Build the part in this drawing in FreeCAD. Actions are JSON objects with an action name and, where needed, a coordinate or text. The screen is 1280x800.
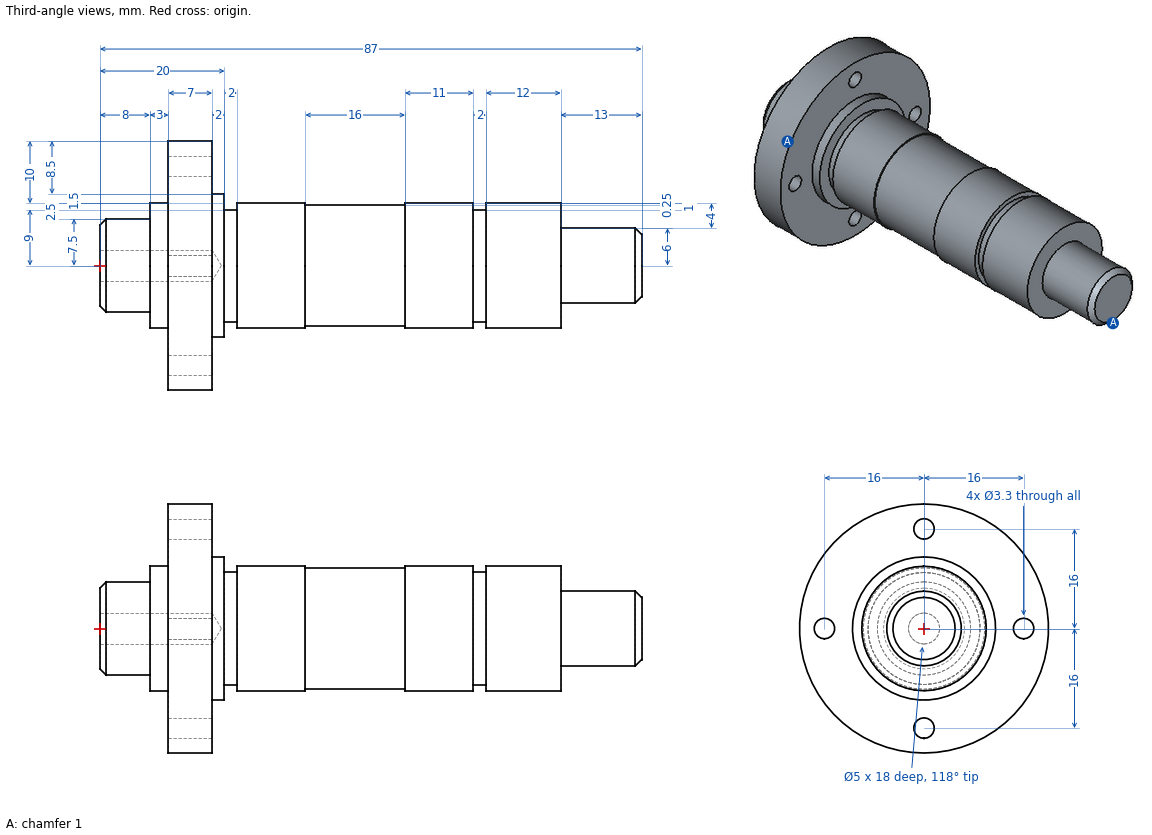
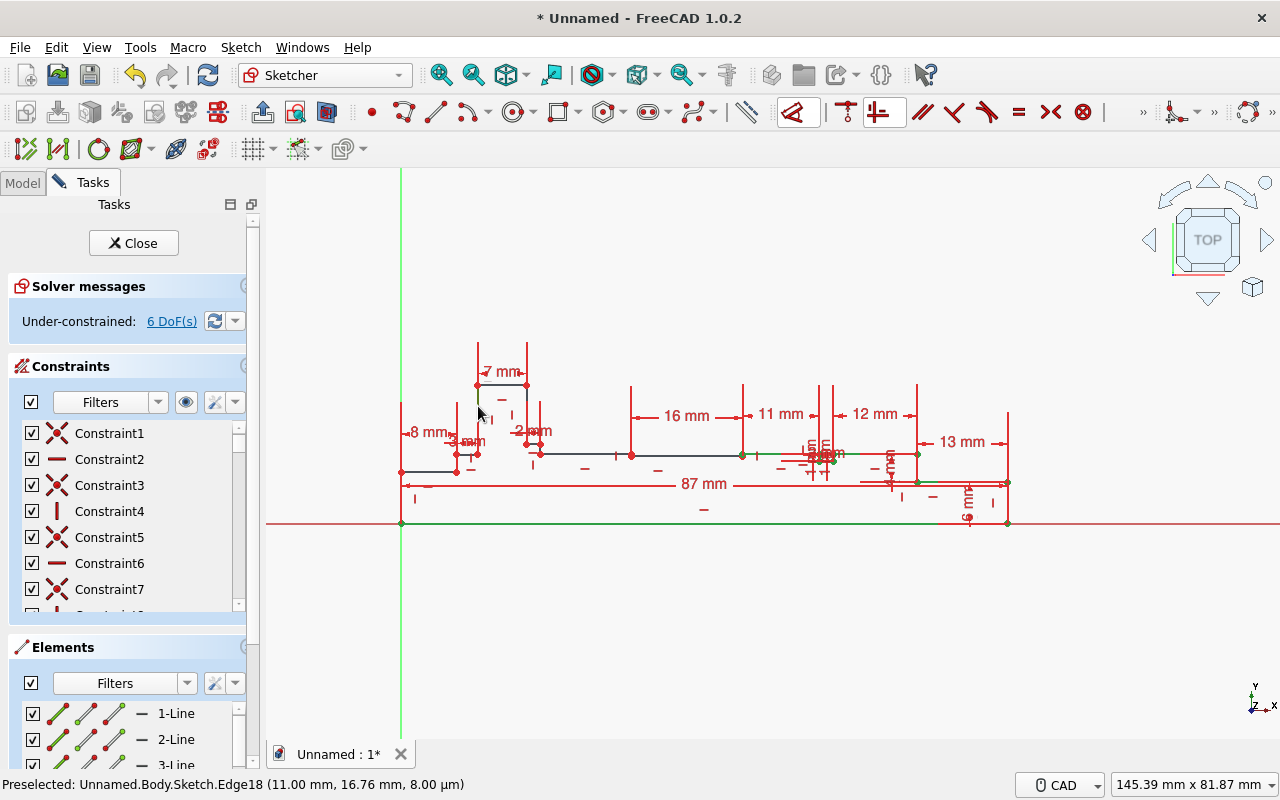
{"action": "key", "text": "i"}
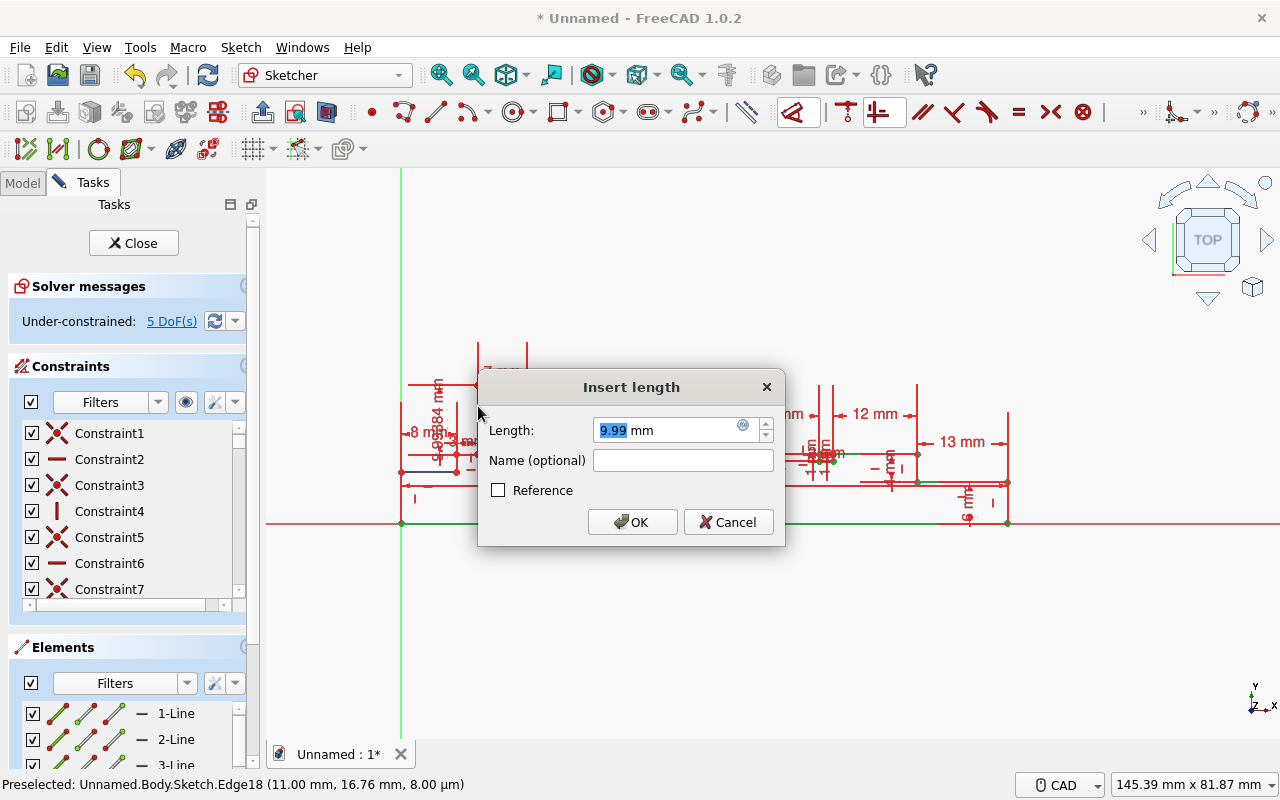
{"action": "type", "text": "10"}
{"action": "key", "text": "Return"}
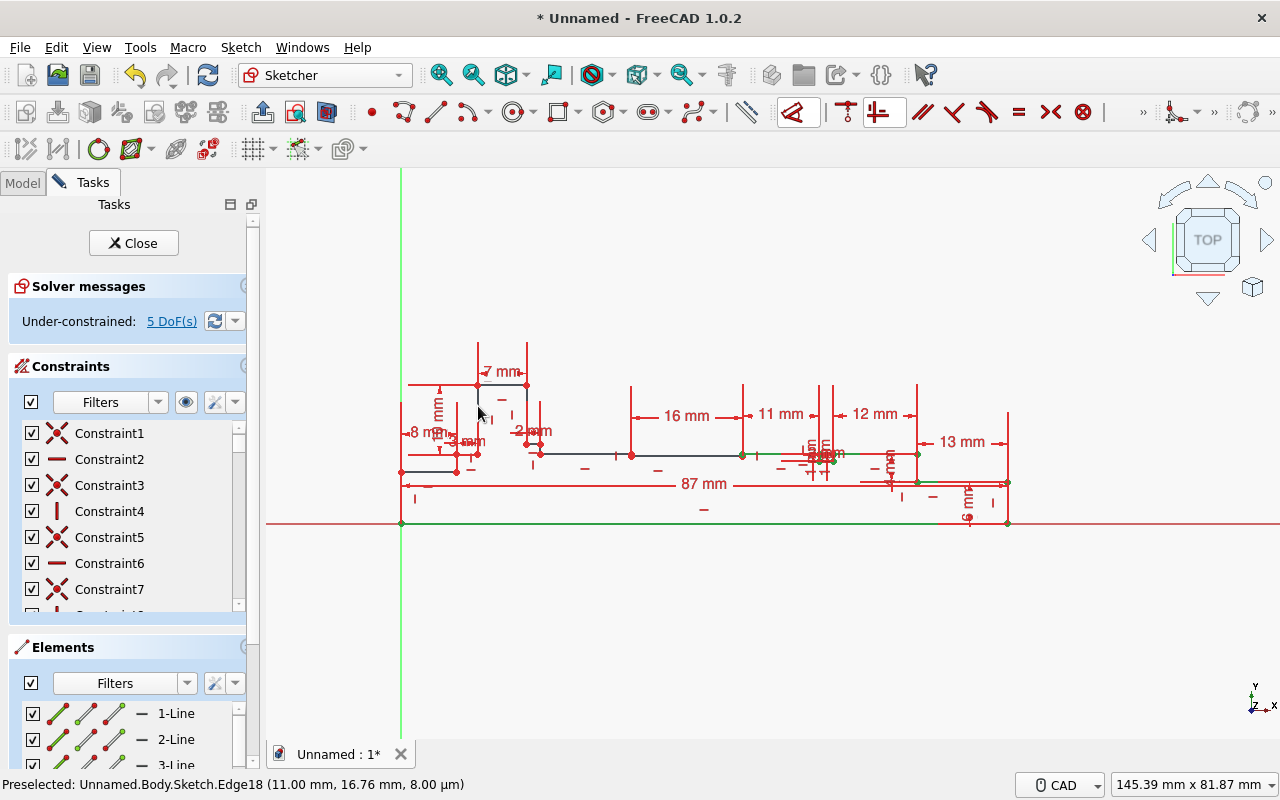
{"action": "scroll", "coordinate": [540, 449], "scroll_direction": "up", "scroll_amount": 7}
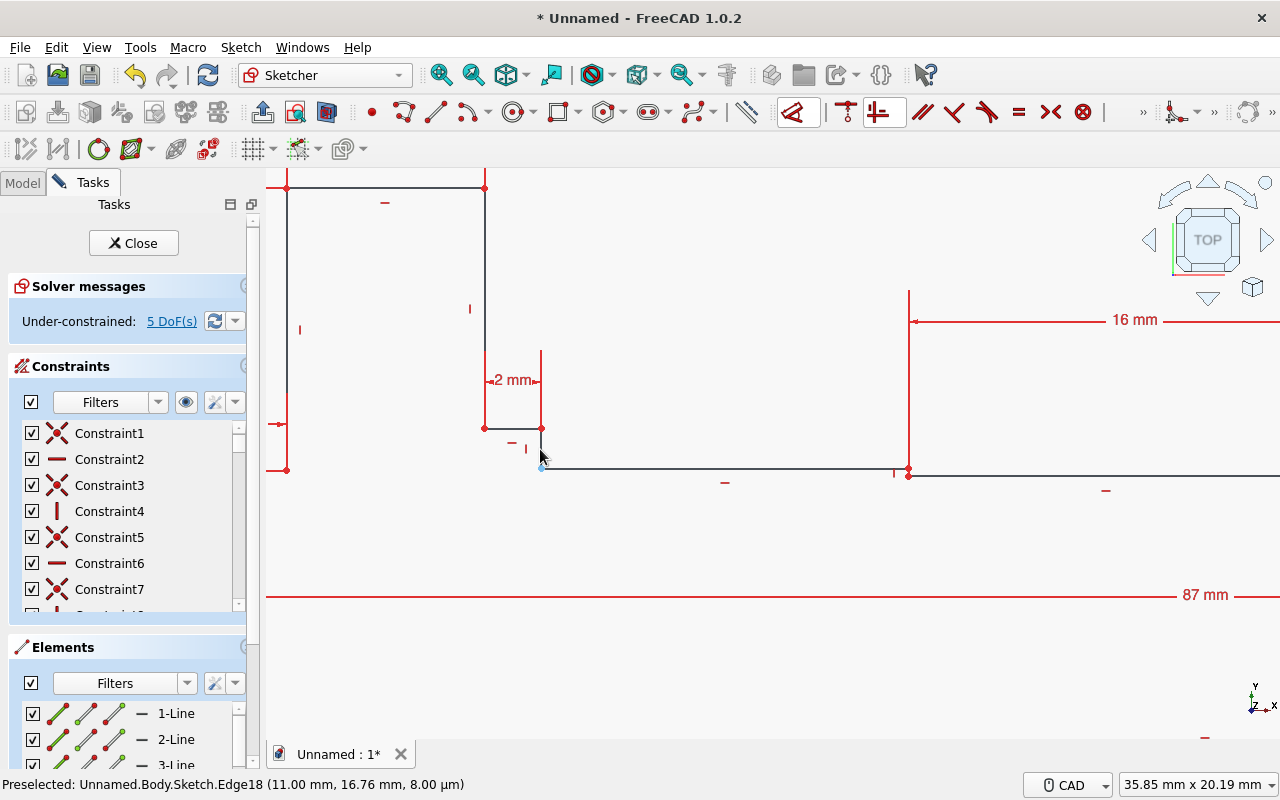
{"action": "left_click", "coordinate": [541, 449]}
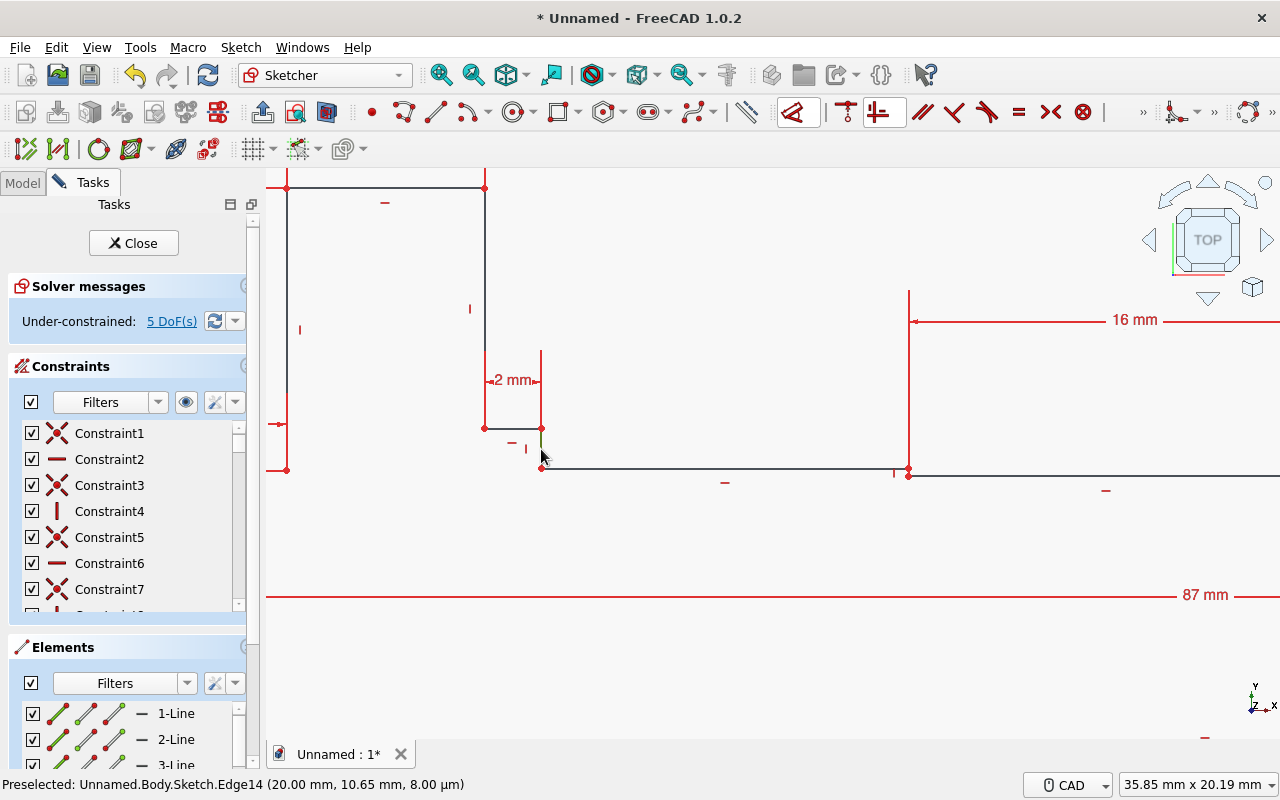
{"action": "key", "text": "i"}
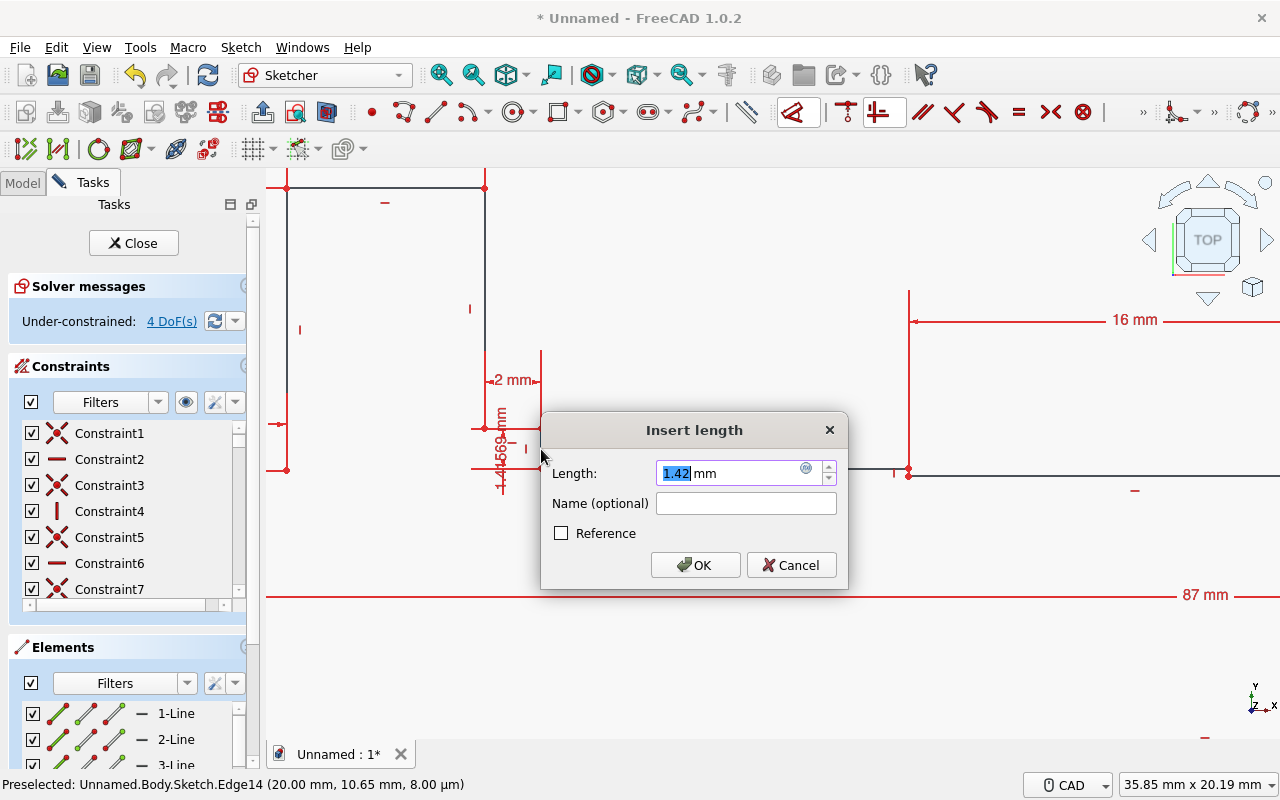
{"action": "type", "text": "1.5"}
{"action": "key", "text": "Return"}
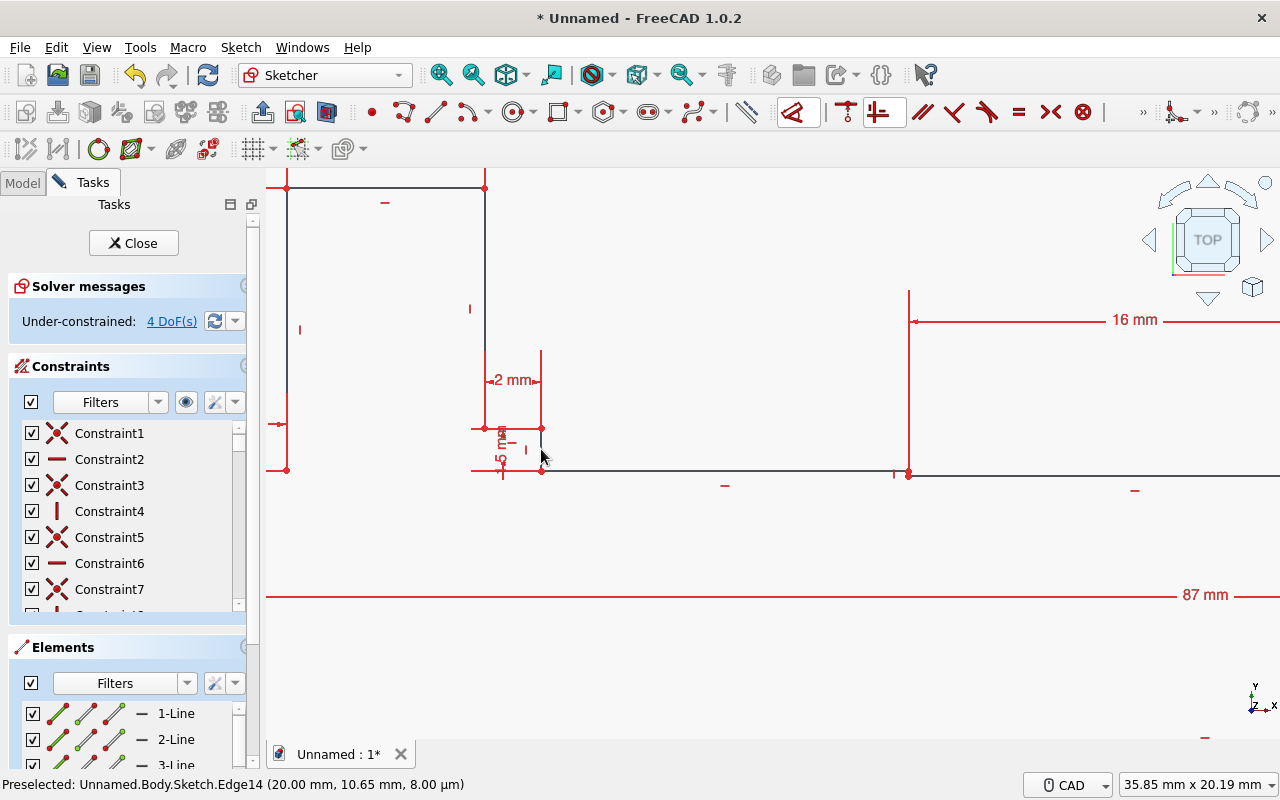
{"action": "scroll", "coordinate": [540, 449], "scroll_direction": "down", "scroll_amount": 7}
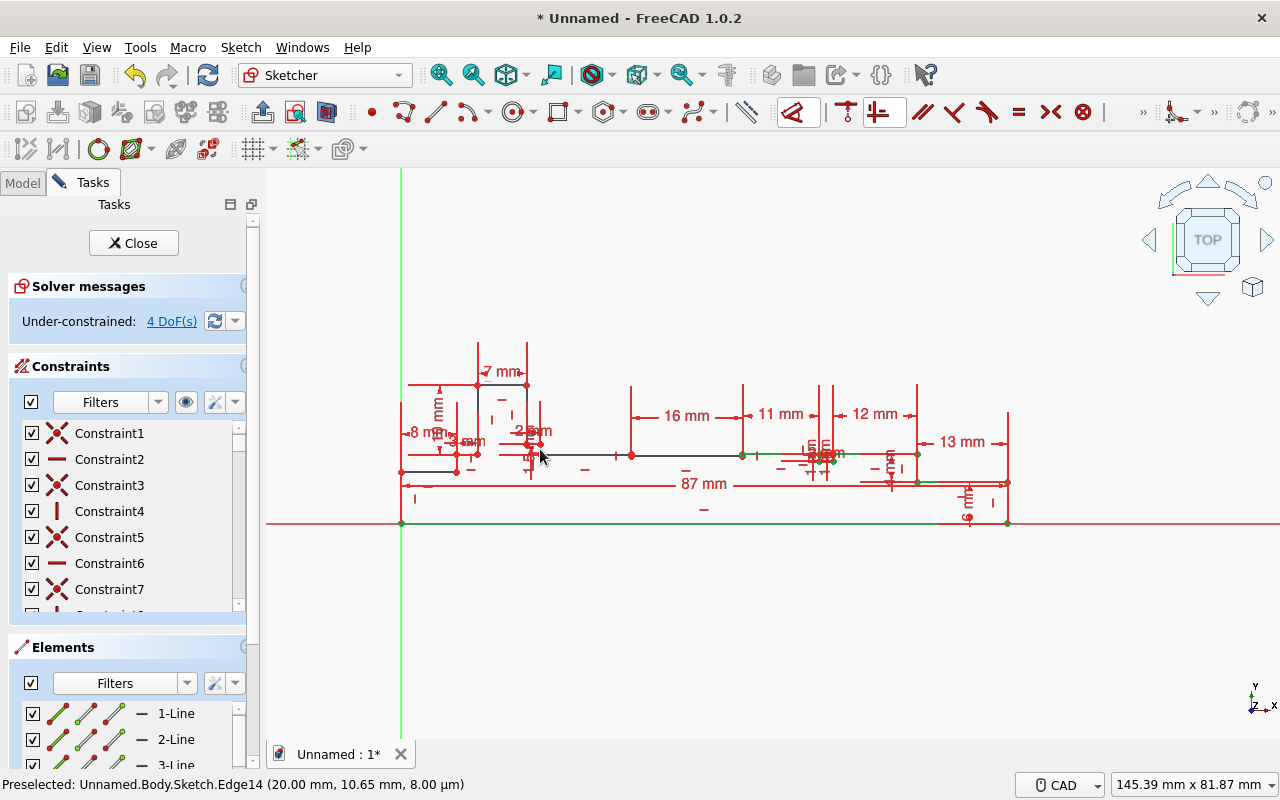
{"action": "left_click", "coordinate": [527, 403]}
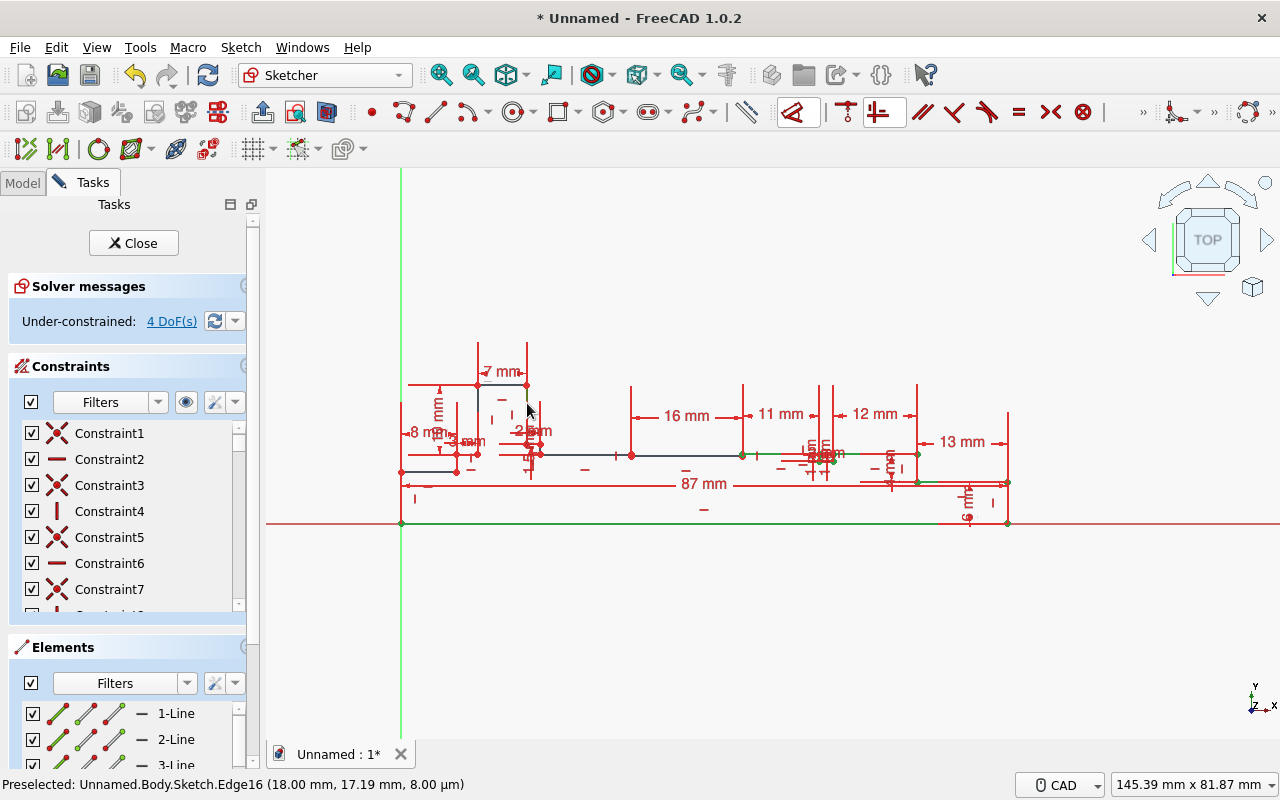
{"action": "key", "text": "i"}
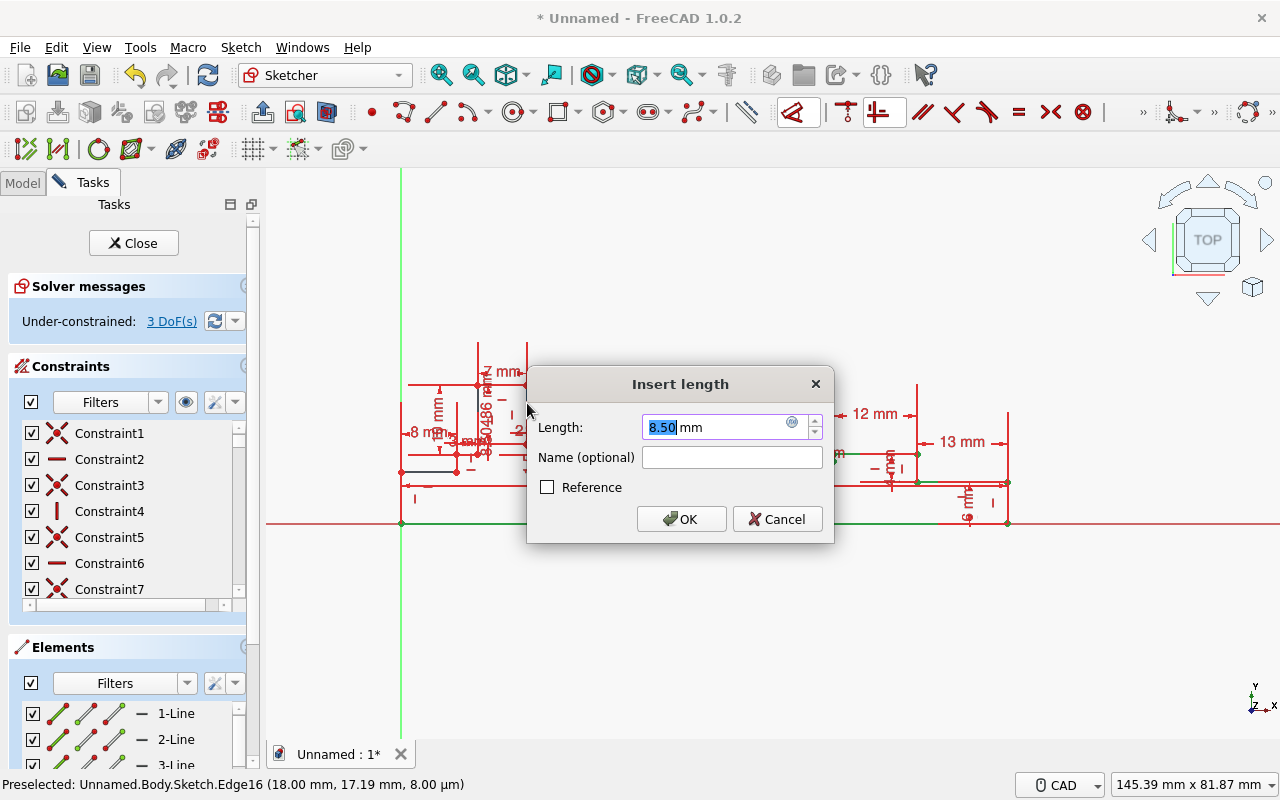
{"action": "type", "text": "8.5"}
{"action": "key", "text": "Return"}